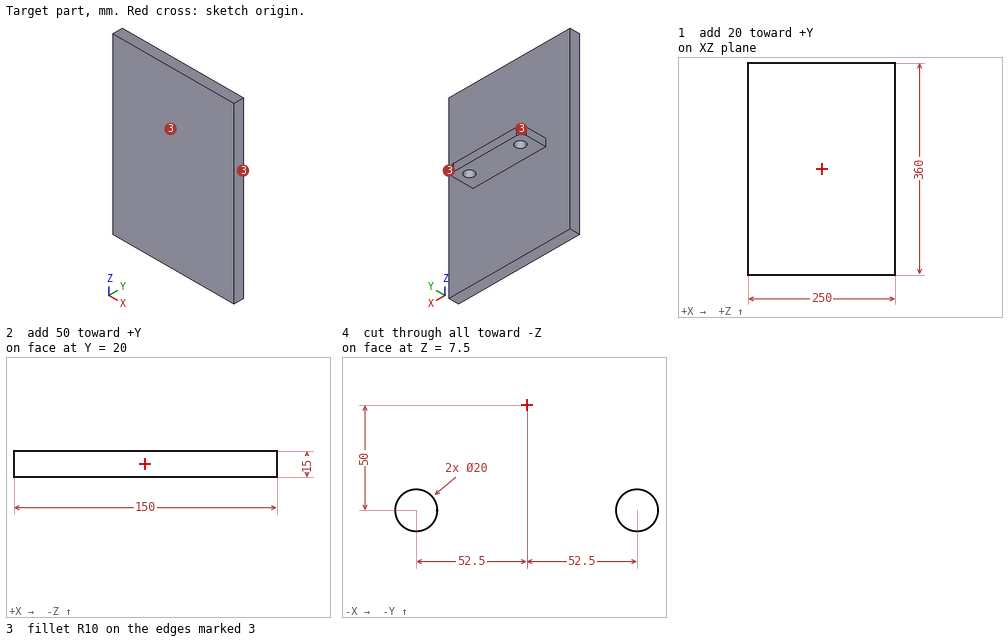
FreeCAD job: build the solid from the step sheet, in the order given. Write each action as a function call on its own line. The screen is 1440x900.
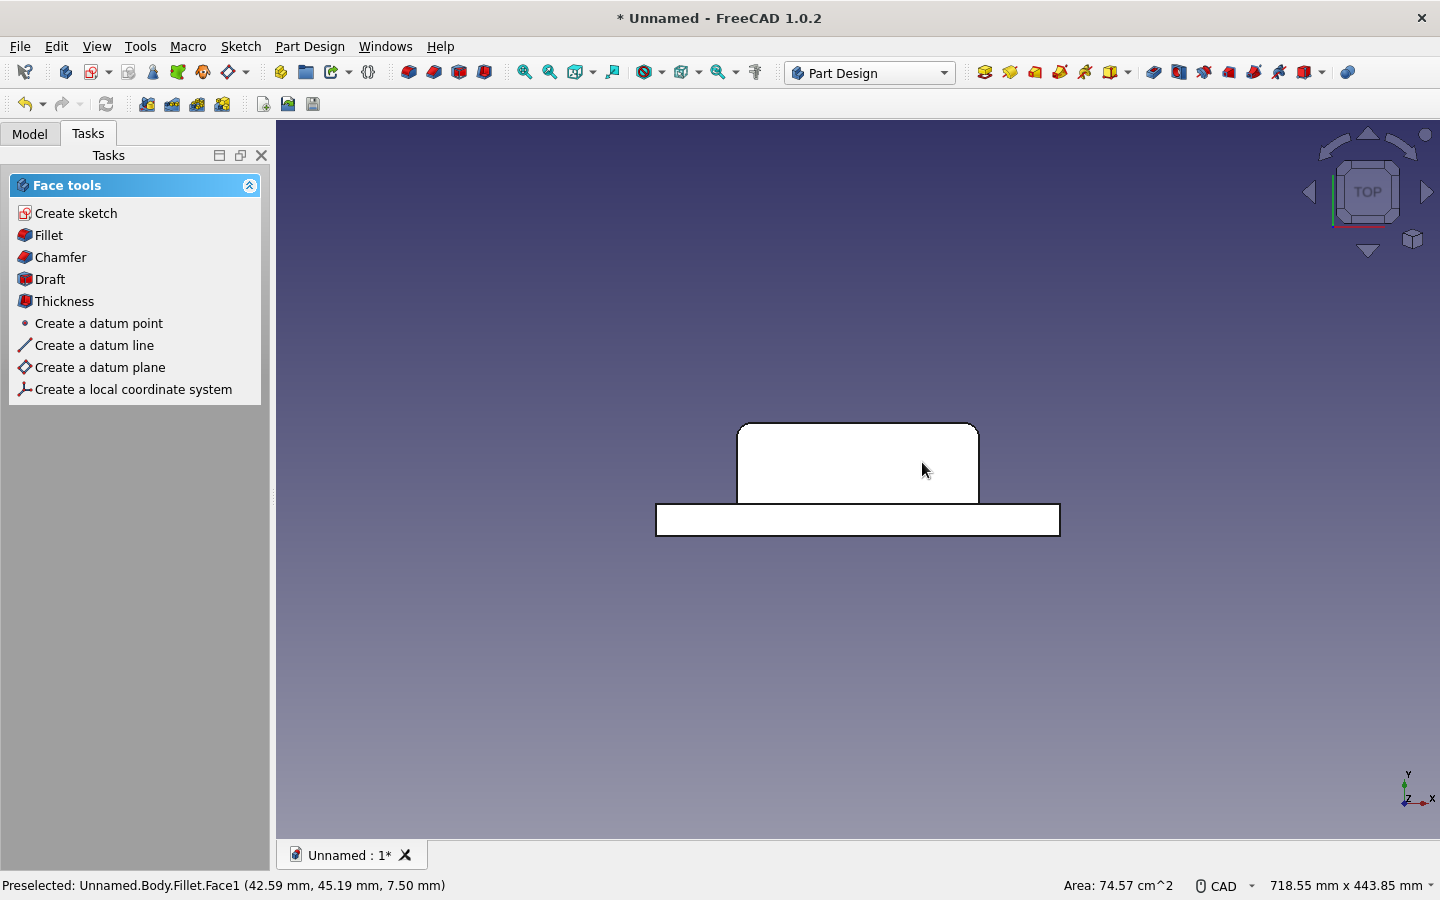
click(90, 72)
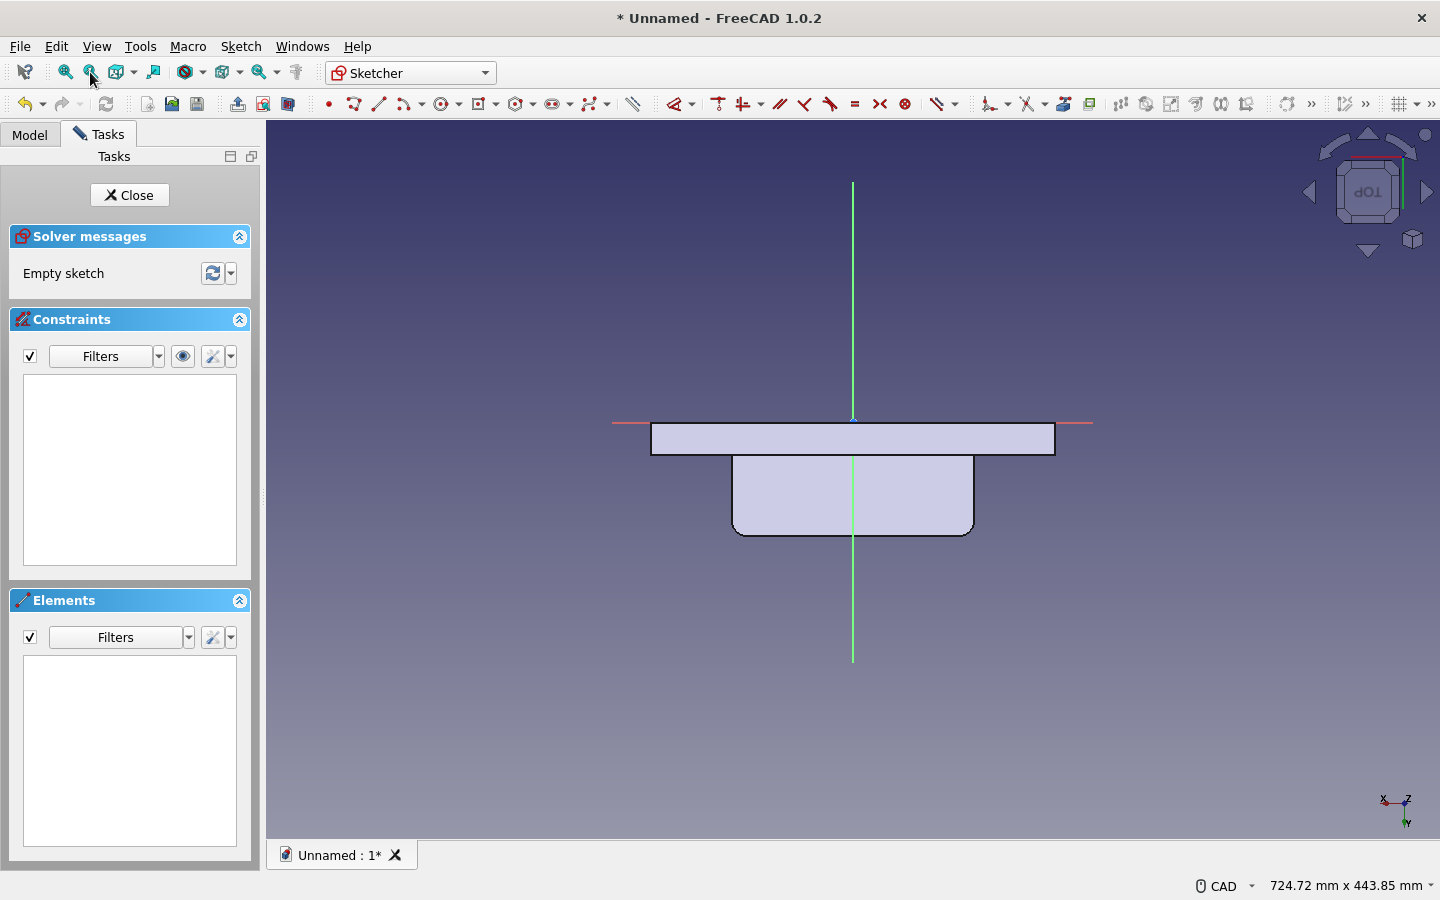
click(288, 104)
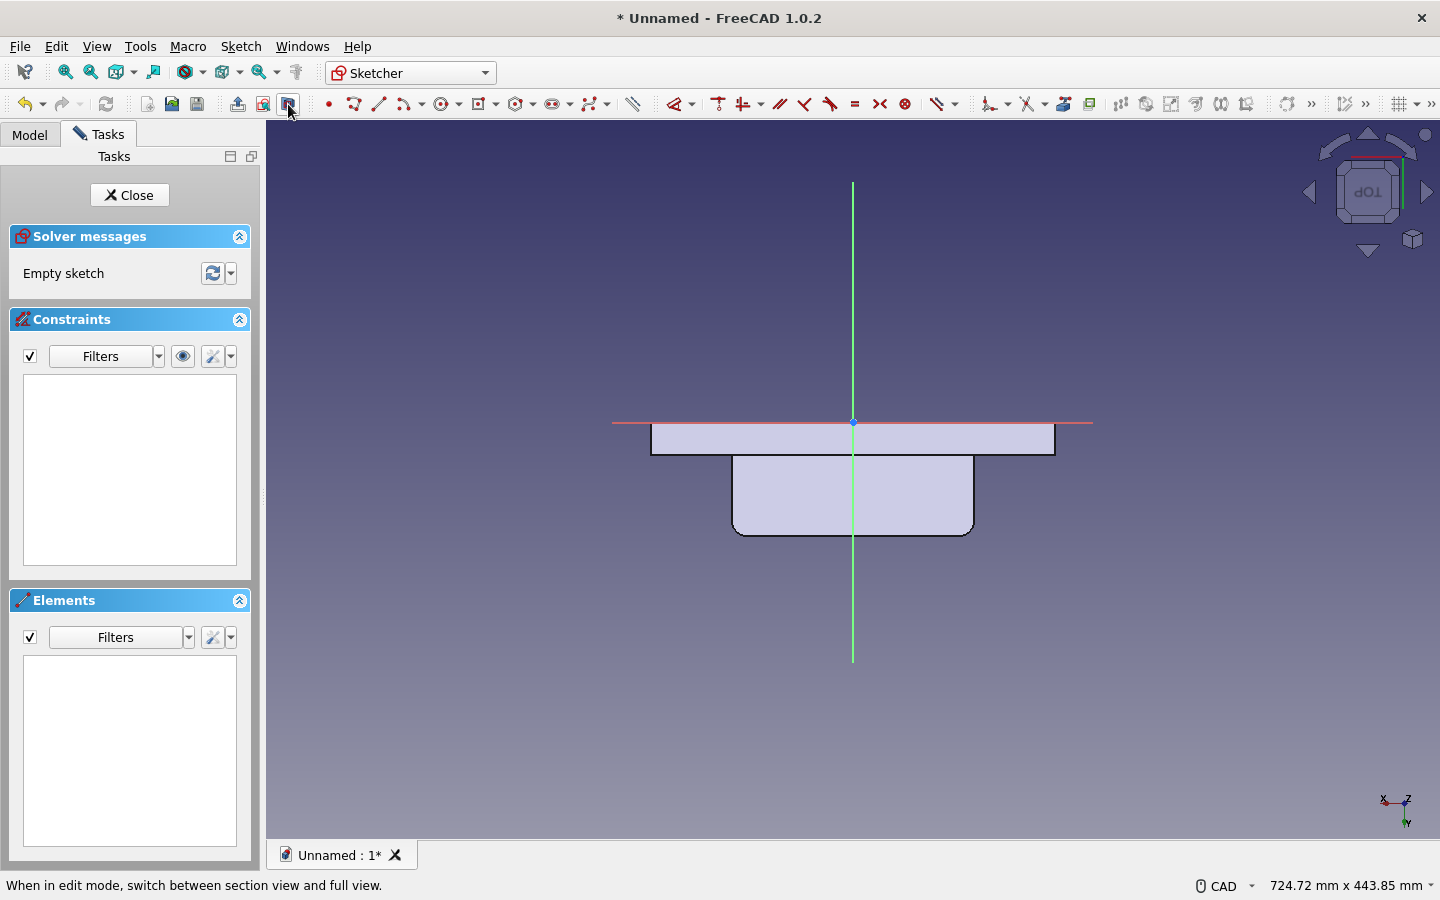
scroll(883, 468, up, 6)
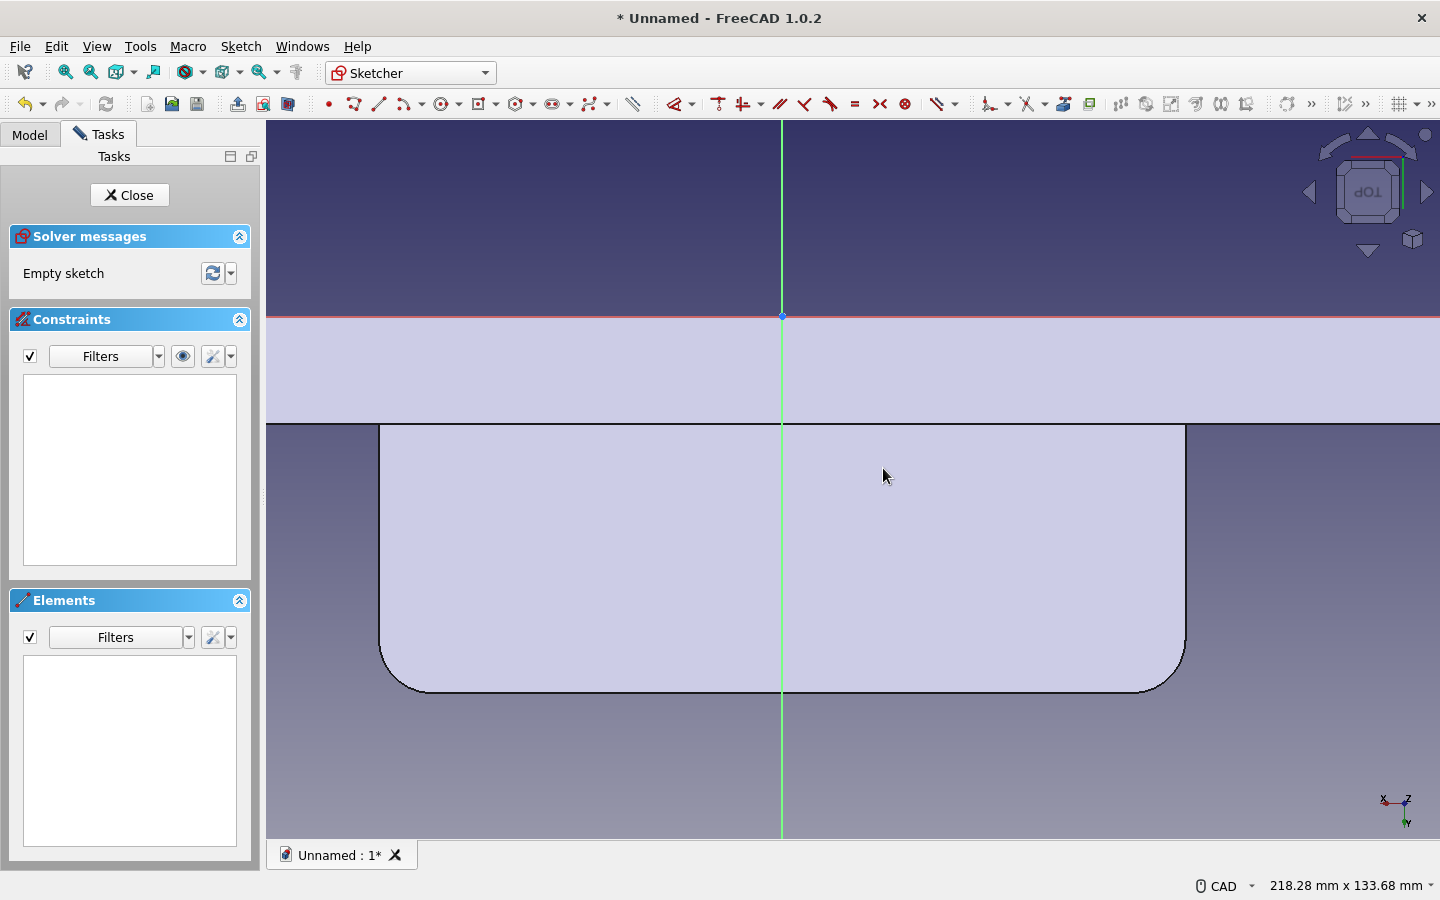
key(g)
key(c)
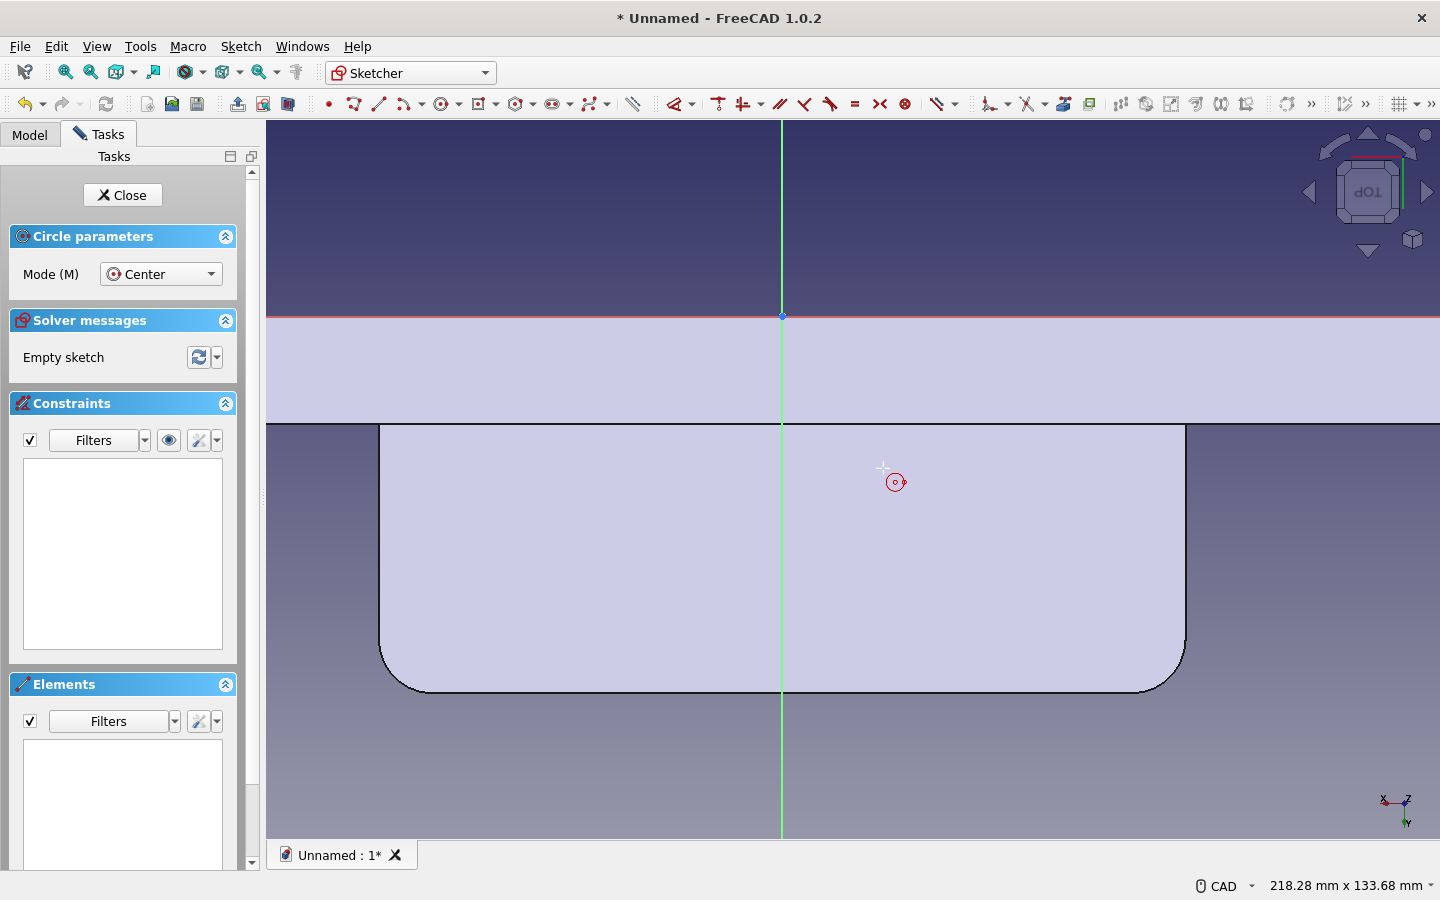
click(500, 586)
click(538, 548)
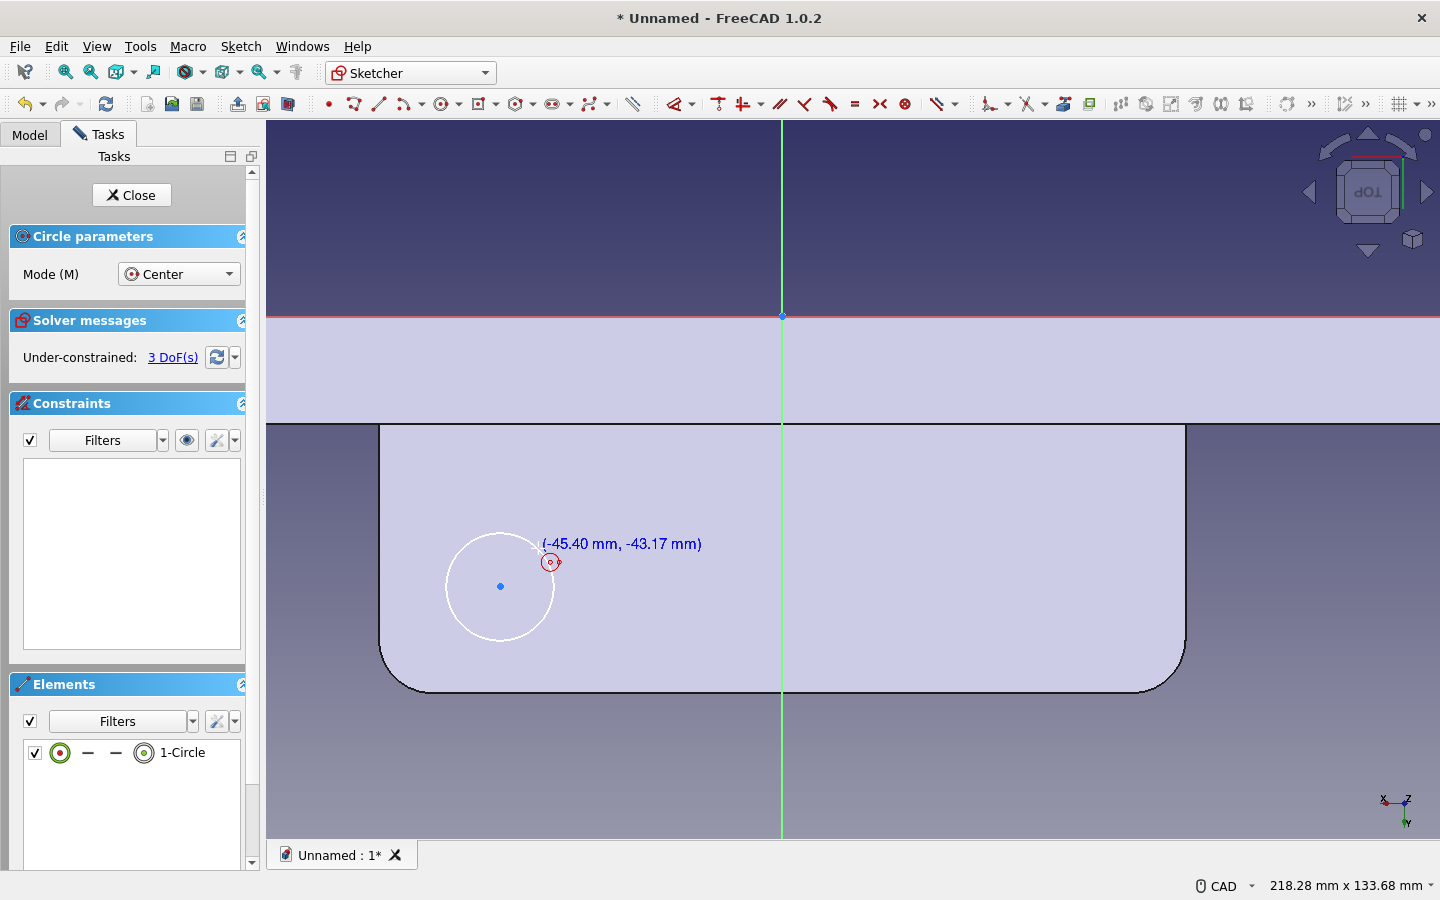
click(1065, 586)
click(1103, 548)
key(Escape)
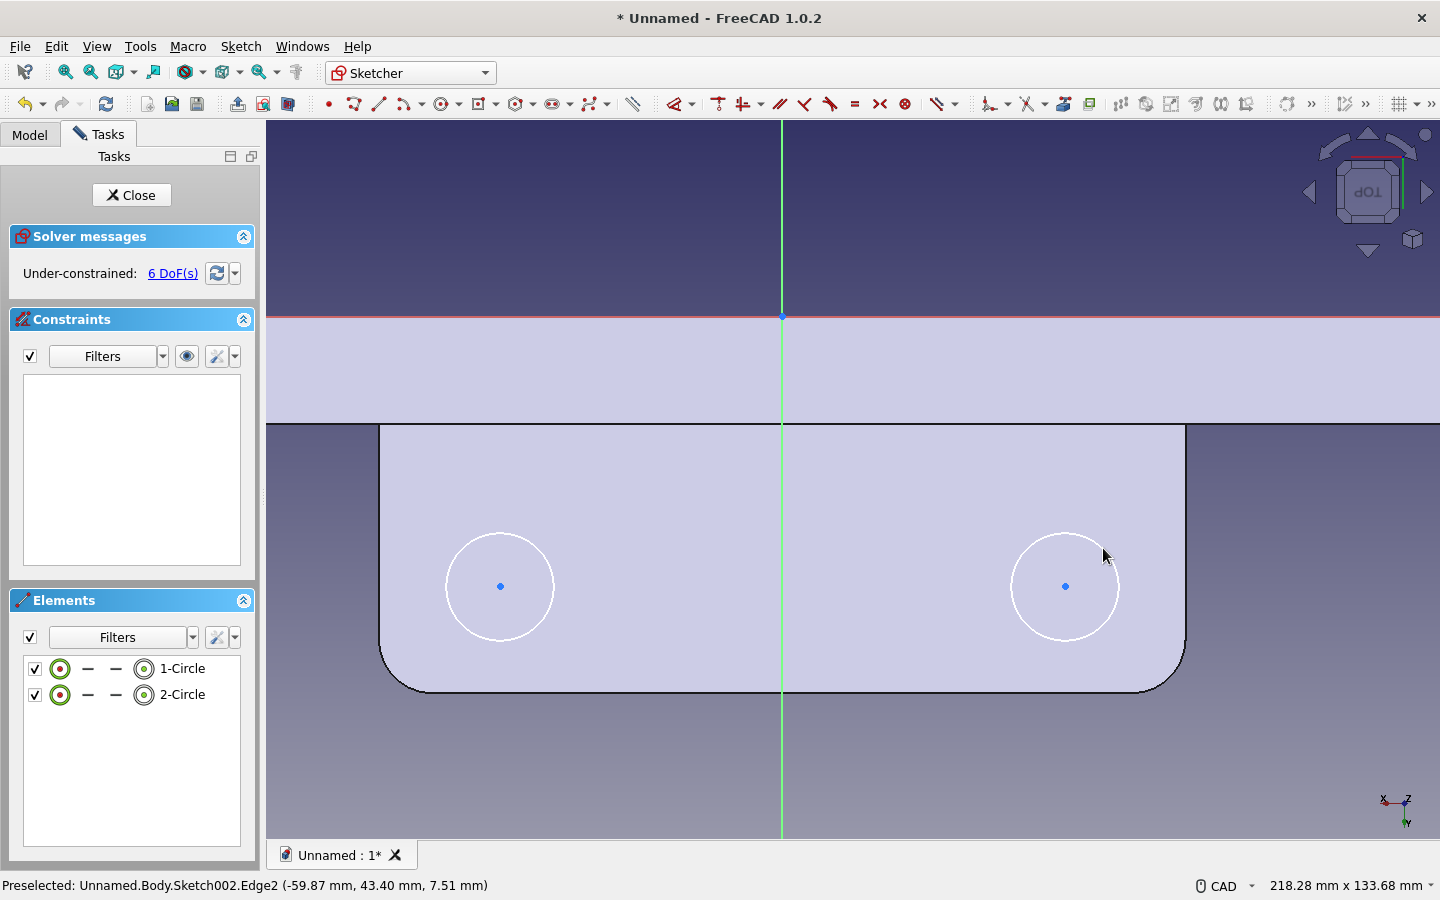
click(538, 549)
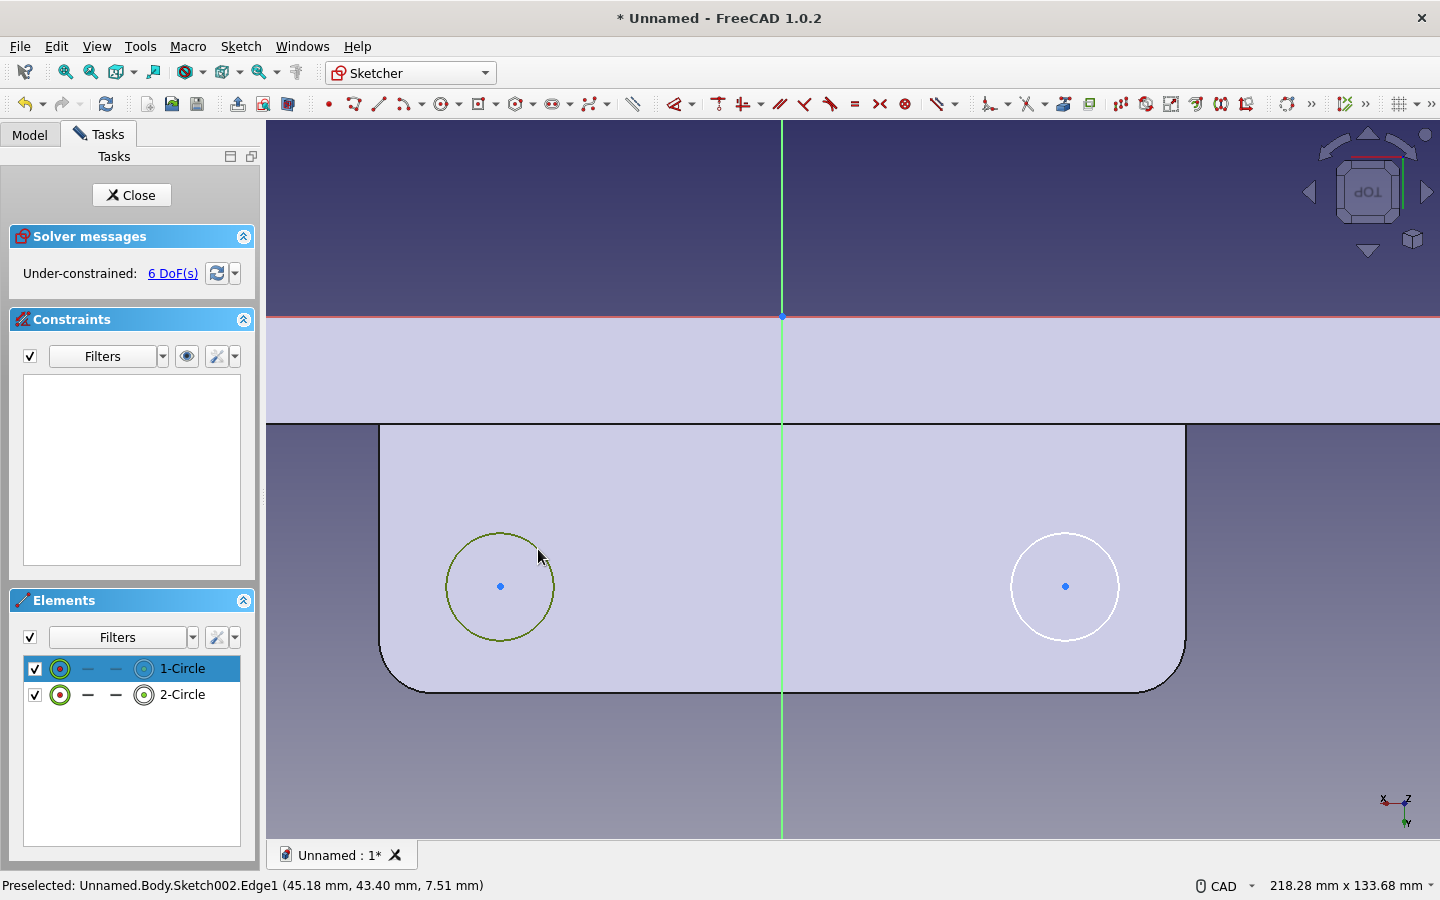
click(1103, 549)